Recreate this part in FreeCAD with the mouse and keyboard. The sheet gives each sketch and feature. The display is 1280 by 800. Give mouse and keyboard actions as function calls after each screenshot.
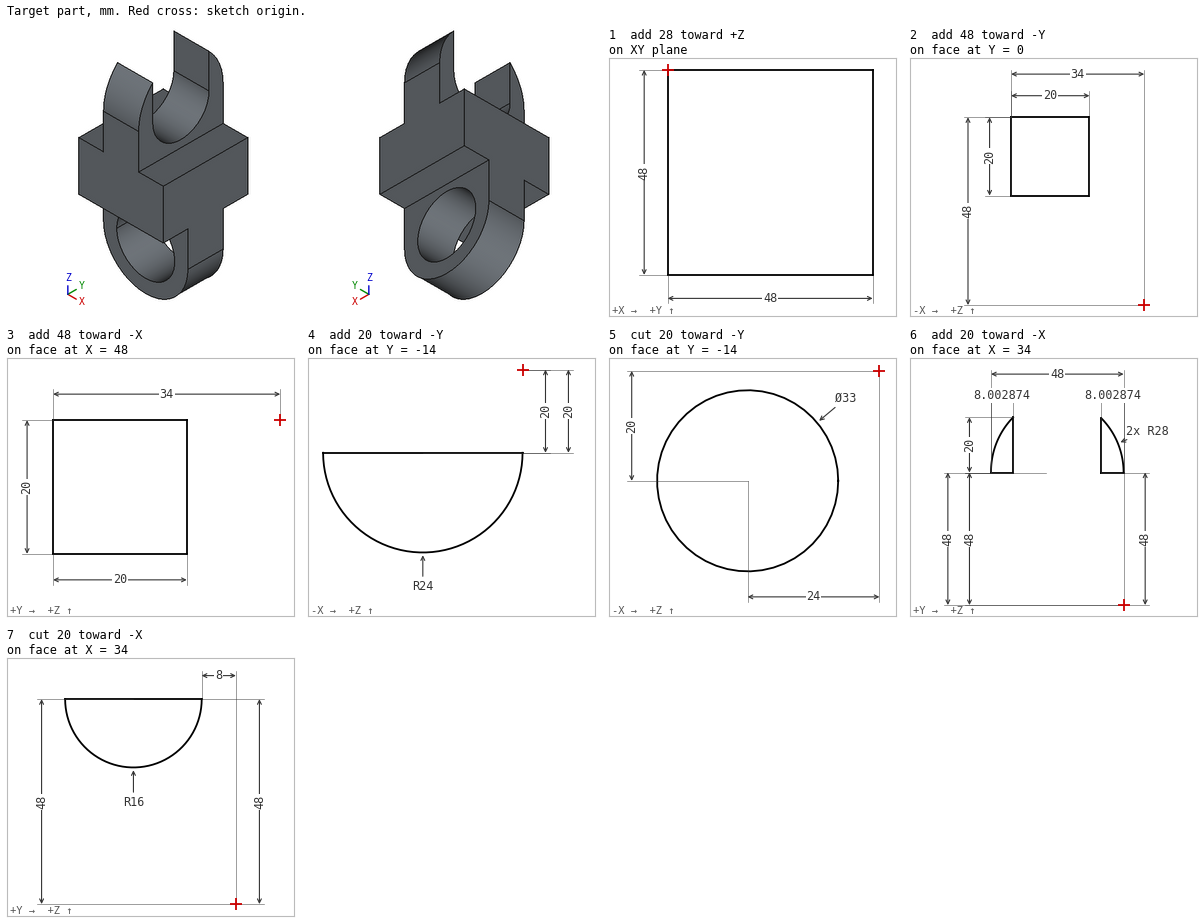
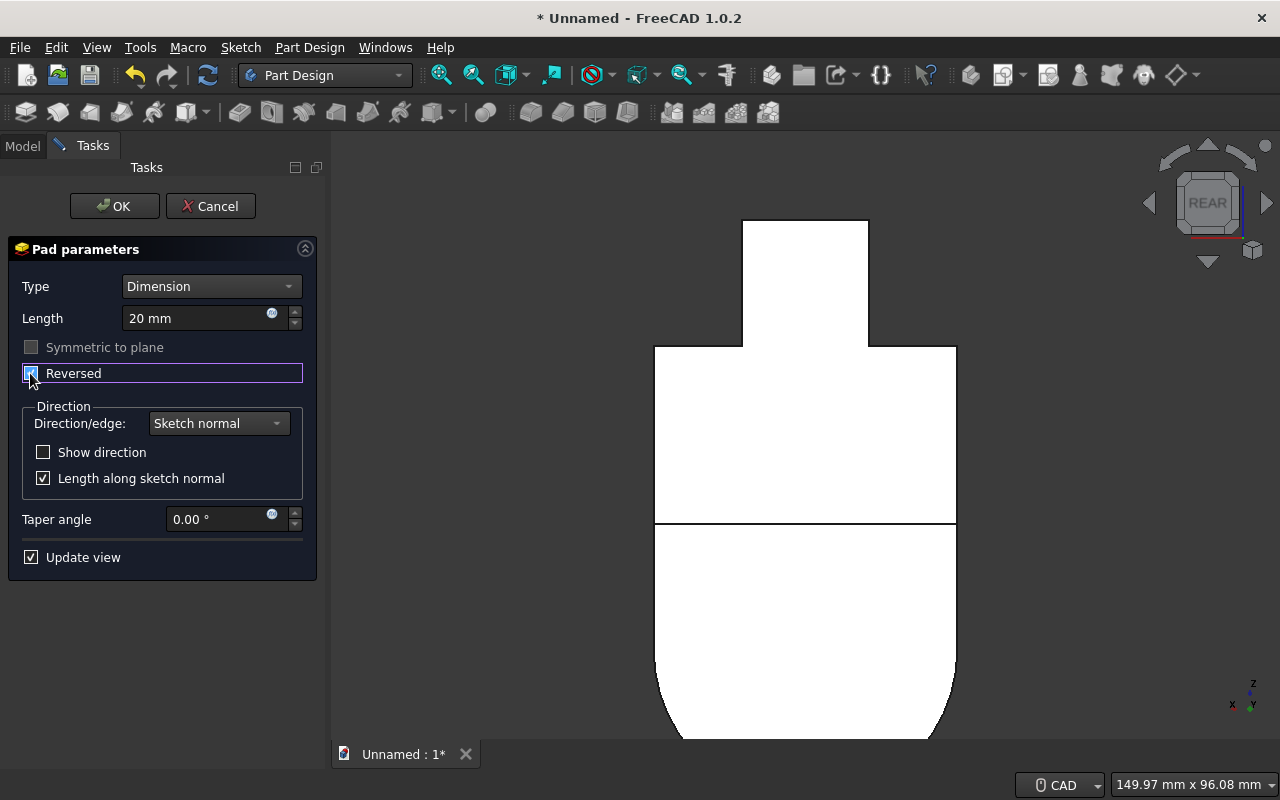
click(115, 206)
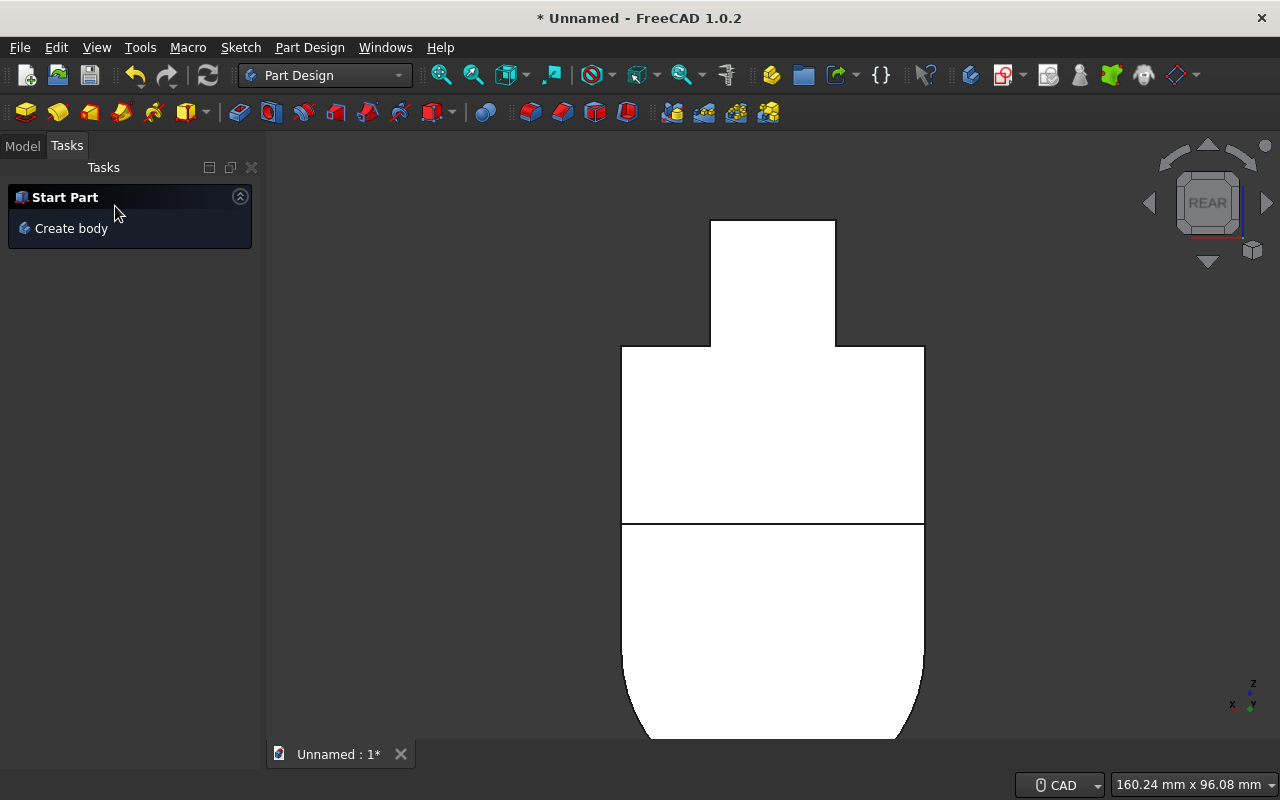
key(v)
key(f)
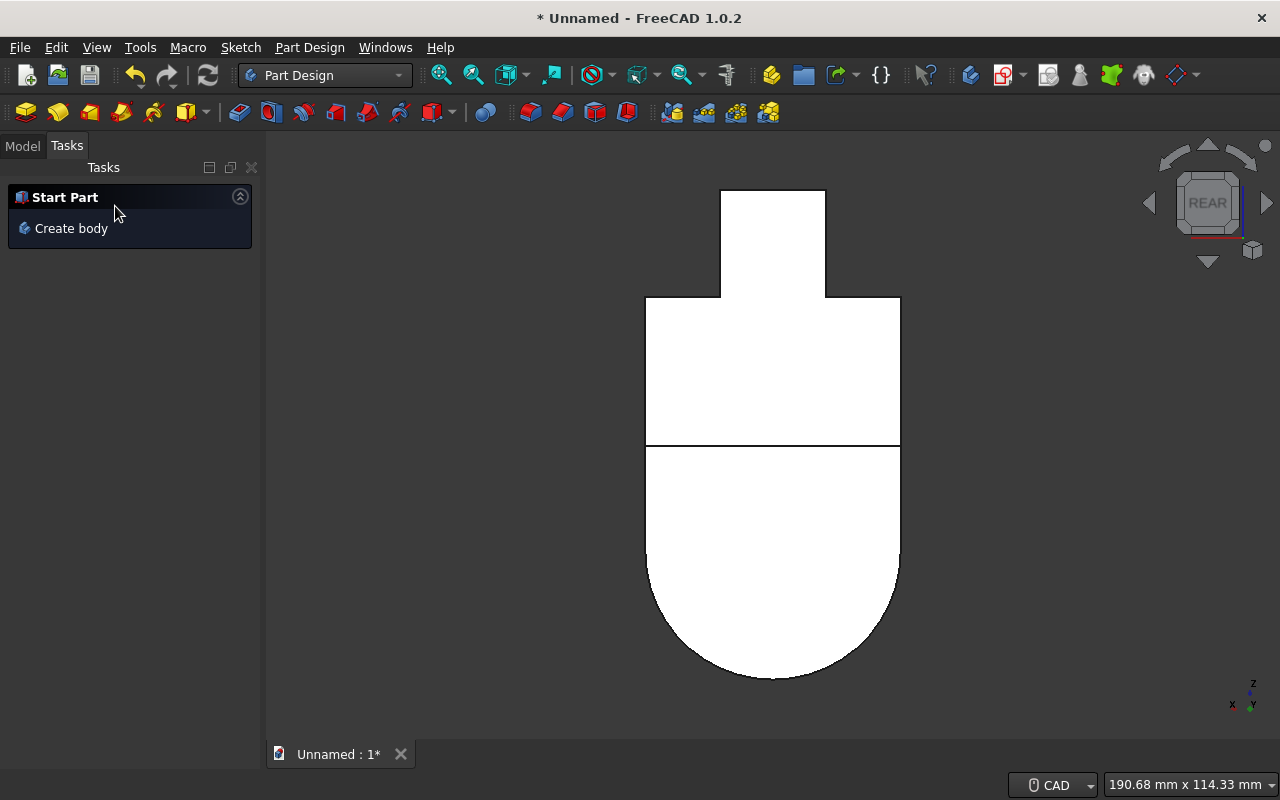
click(773, 562)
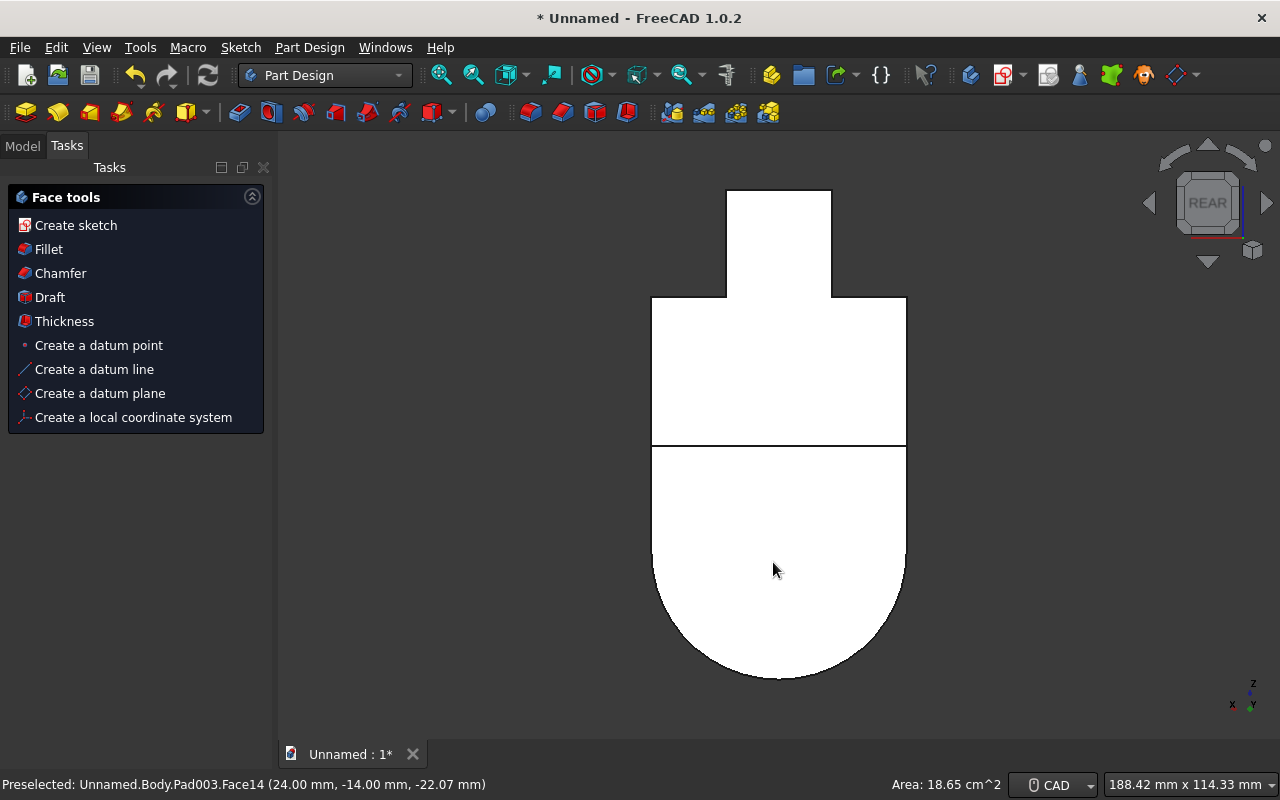
click(1004, 76)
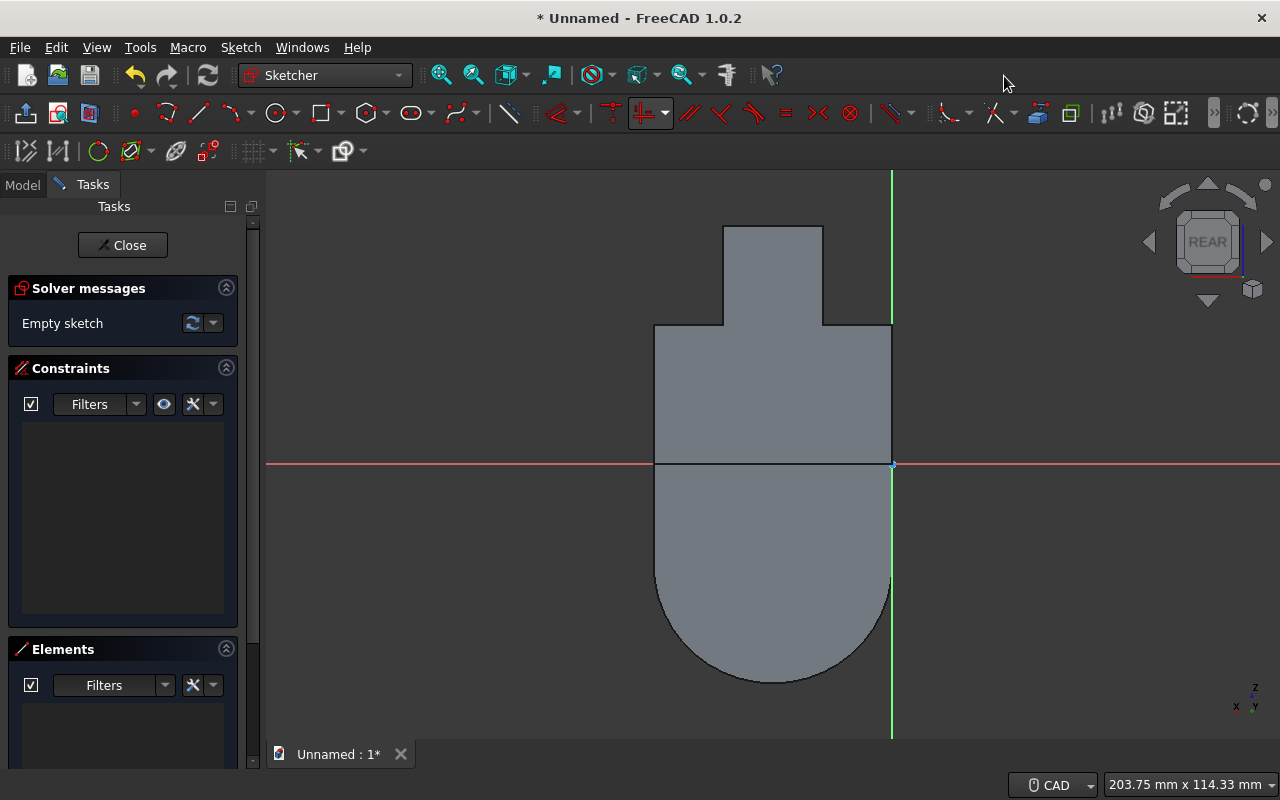
key(q)
key(s)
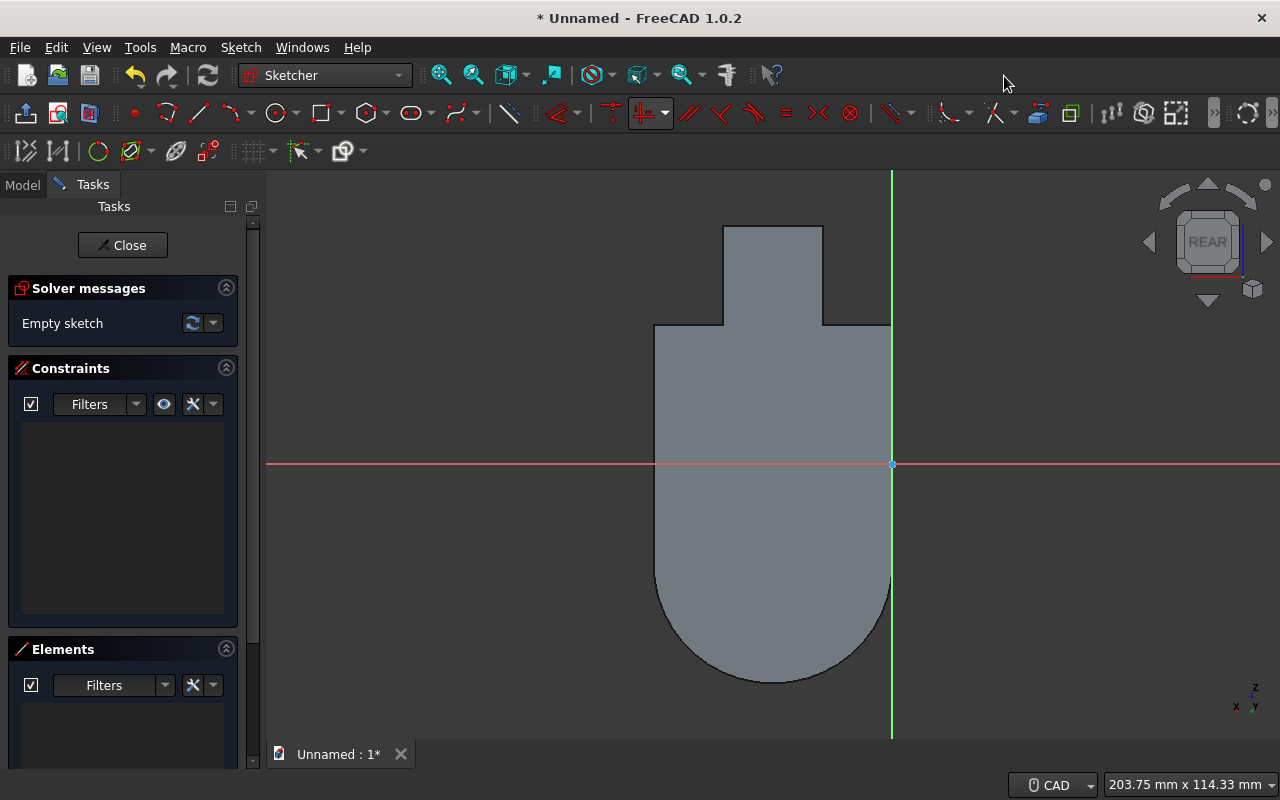
scroll(898, 678, up, 3)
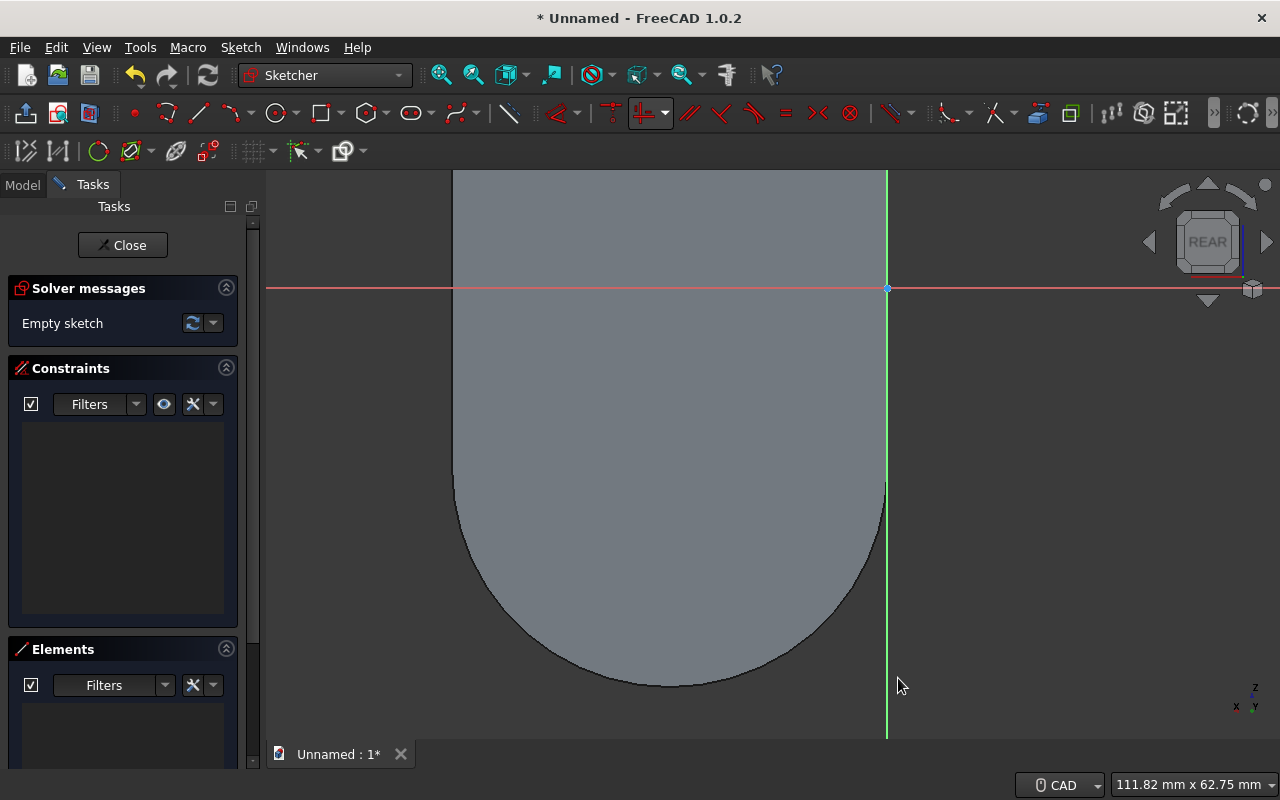
key(g)
key(c)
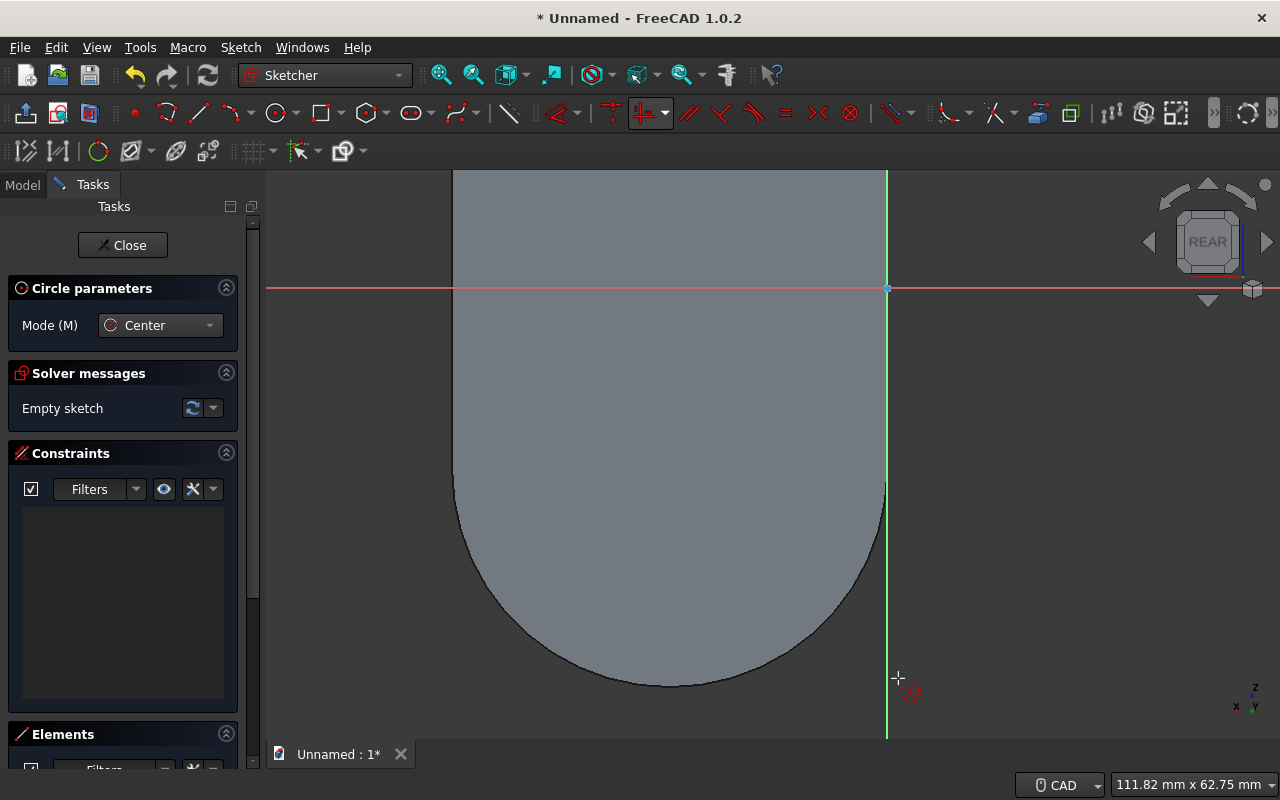
click(670, 470)
click(776, 364)
key(Escape)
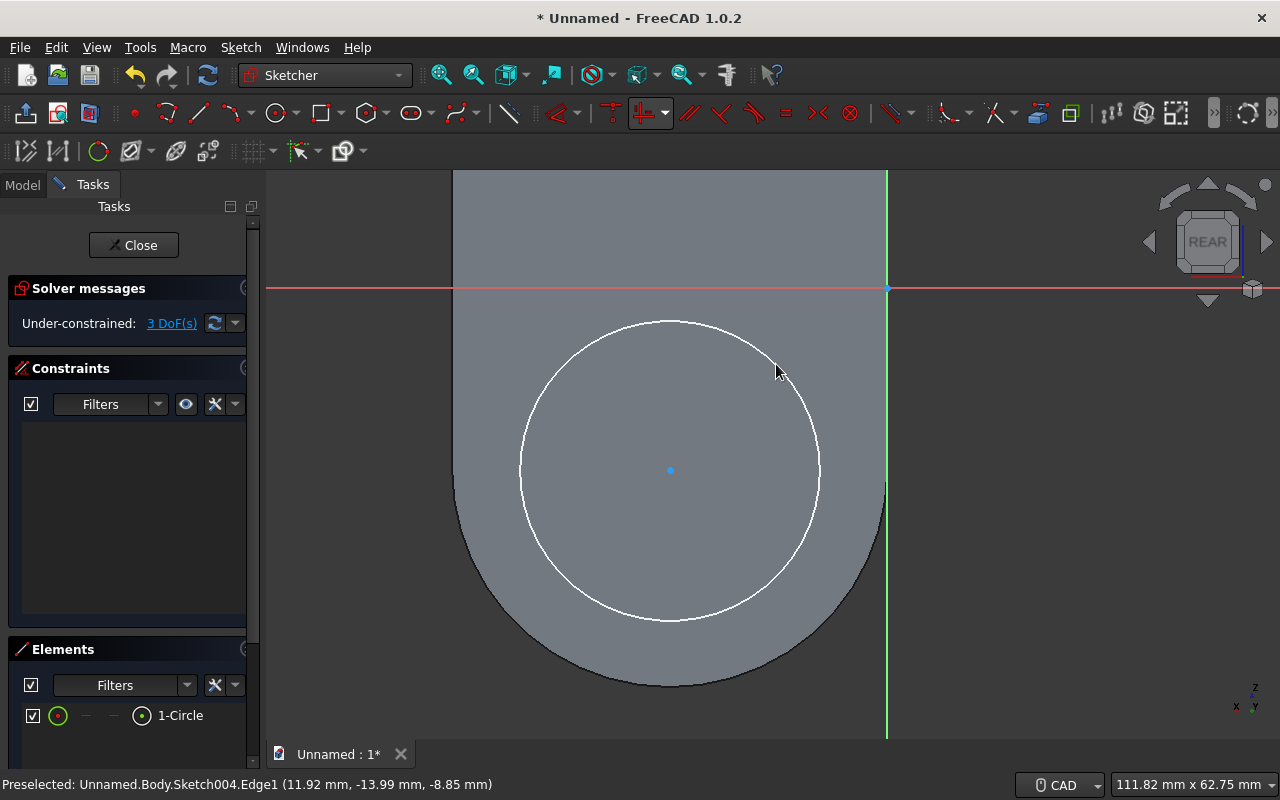
key(d)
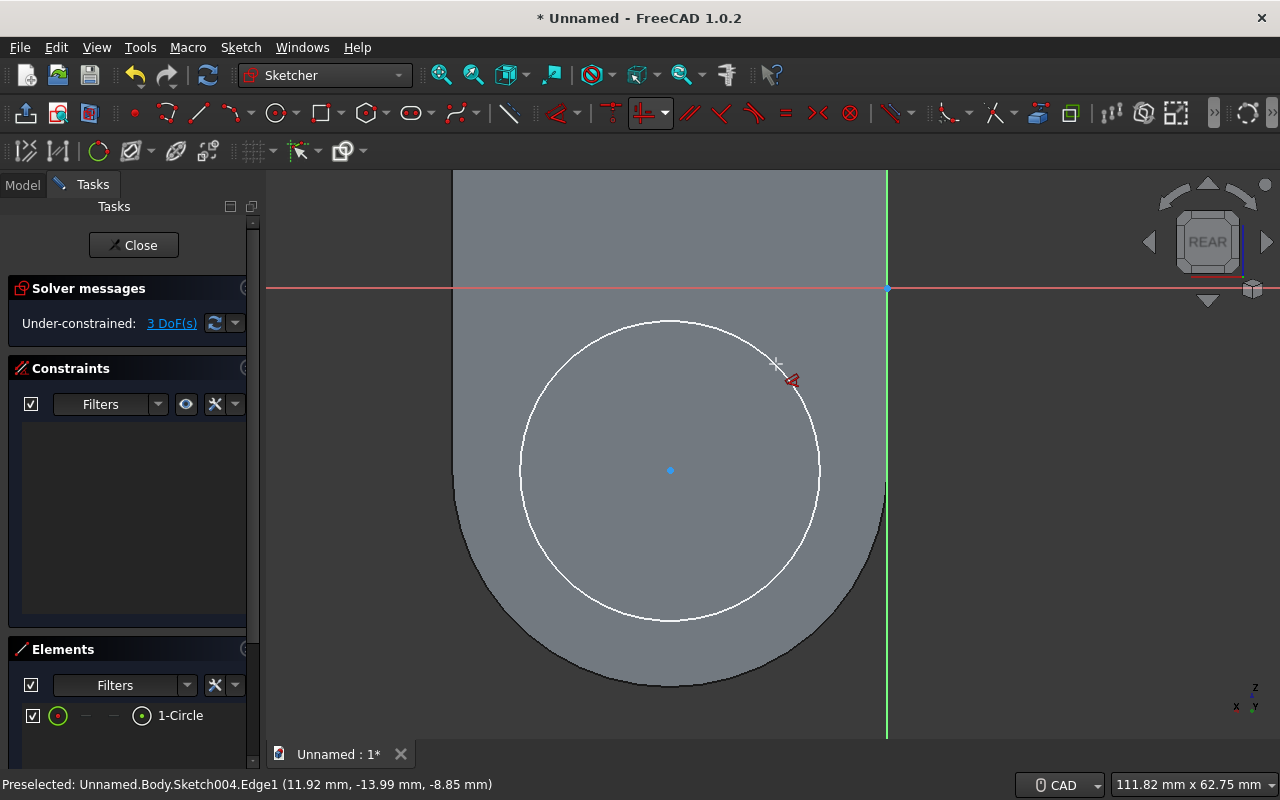
click(776, 365)
click(799, 342)